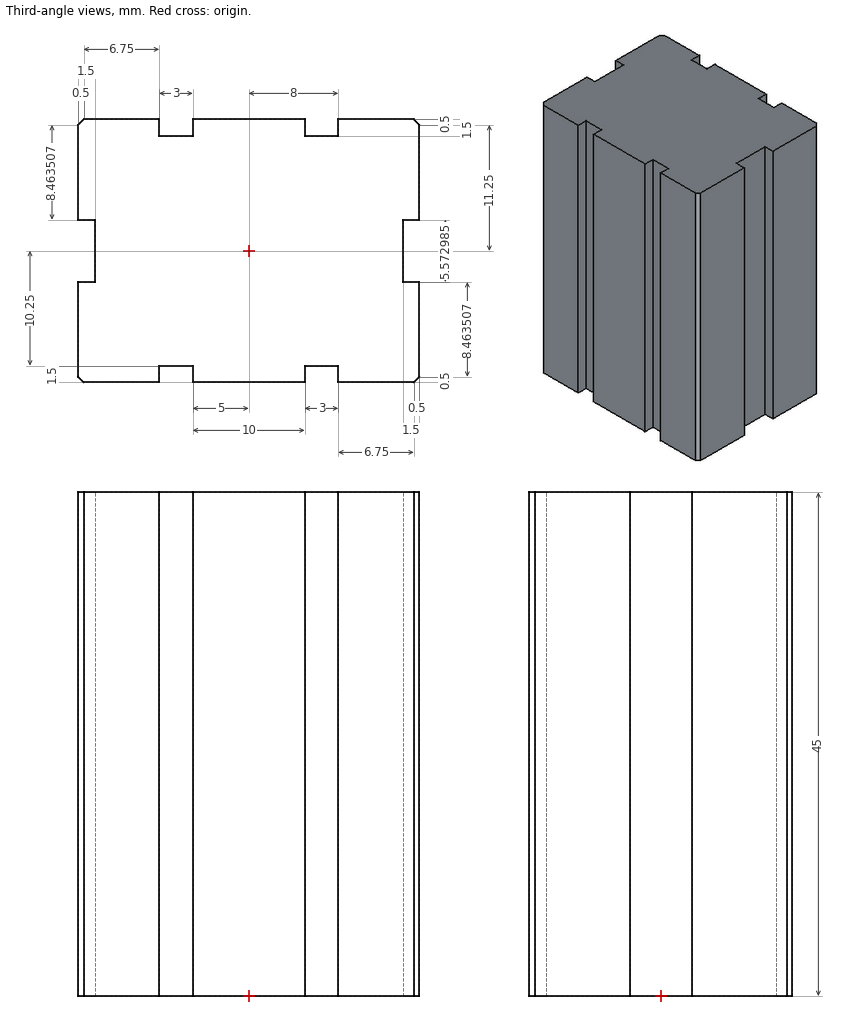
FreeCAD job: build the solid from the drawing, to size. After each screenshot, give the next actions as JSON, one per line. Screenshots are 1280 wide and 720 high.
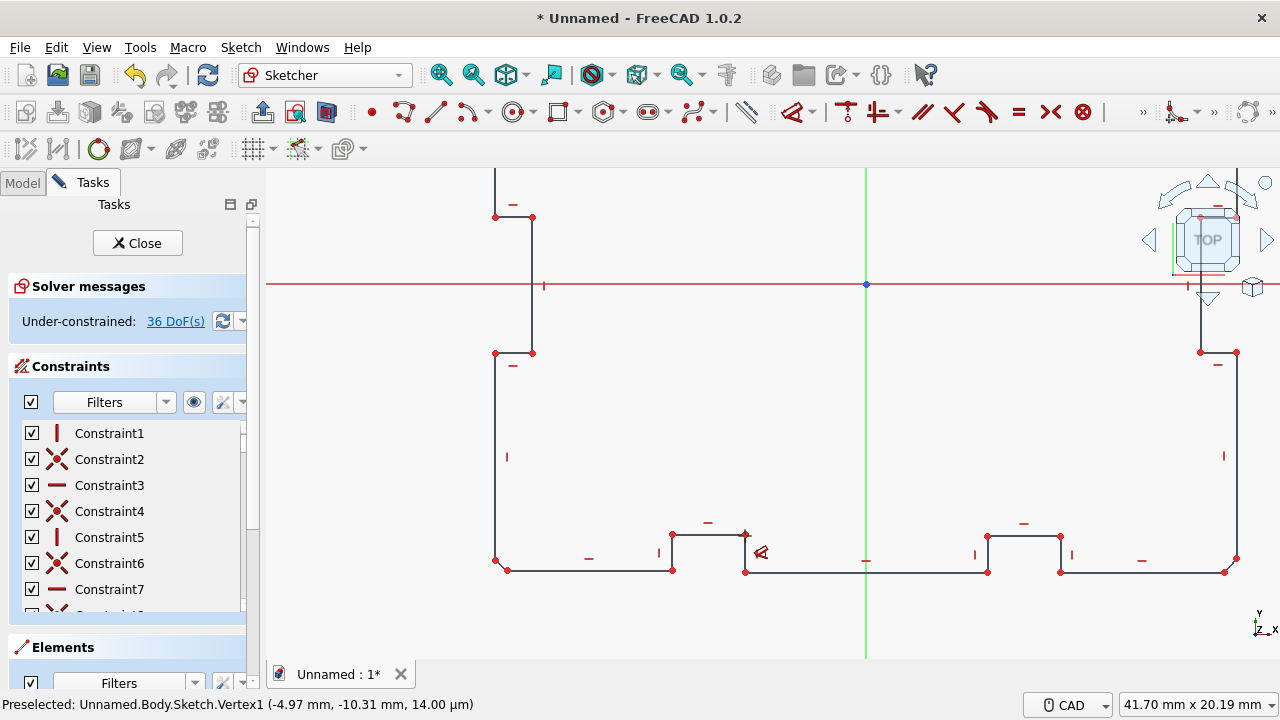
{"action": "left_click", "coordinate": [1010, 536]}
{"action": "left_click", "coordinate": [1024, 570]}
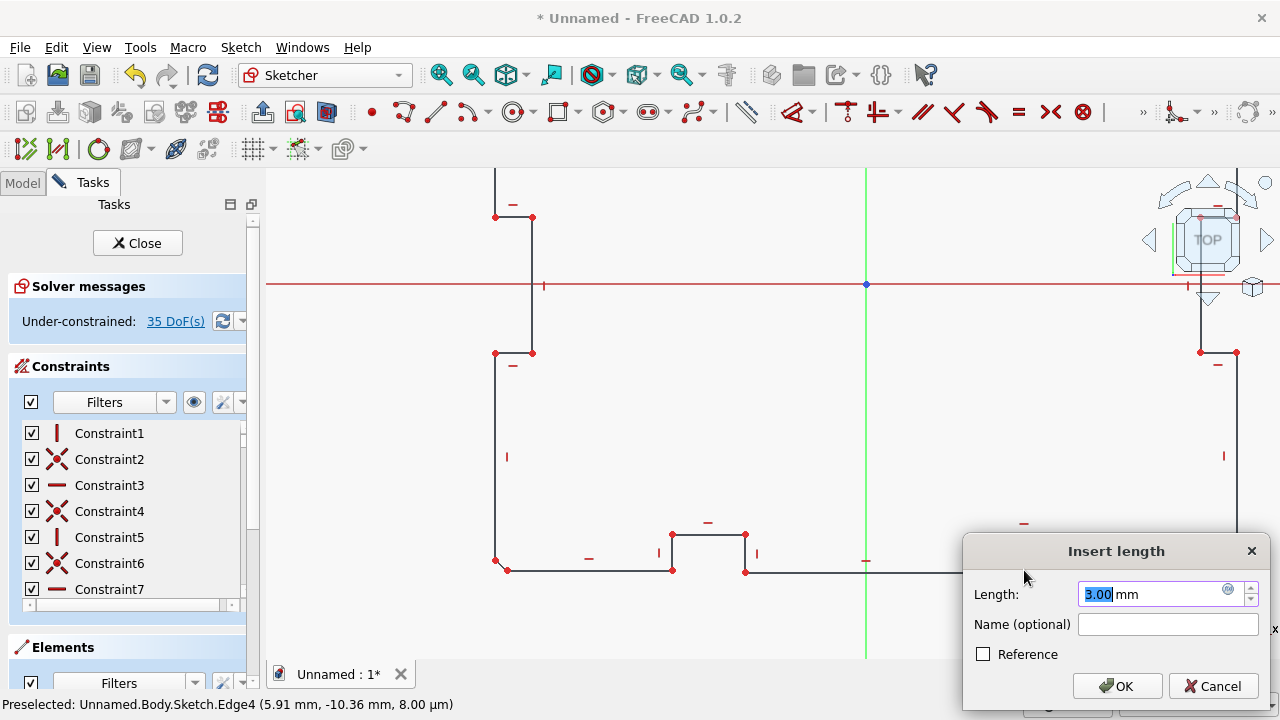
{"action": "type", "text": "3"}
{"action": "key", "text": "Return"}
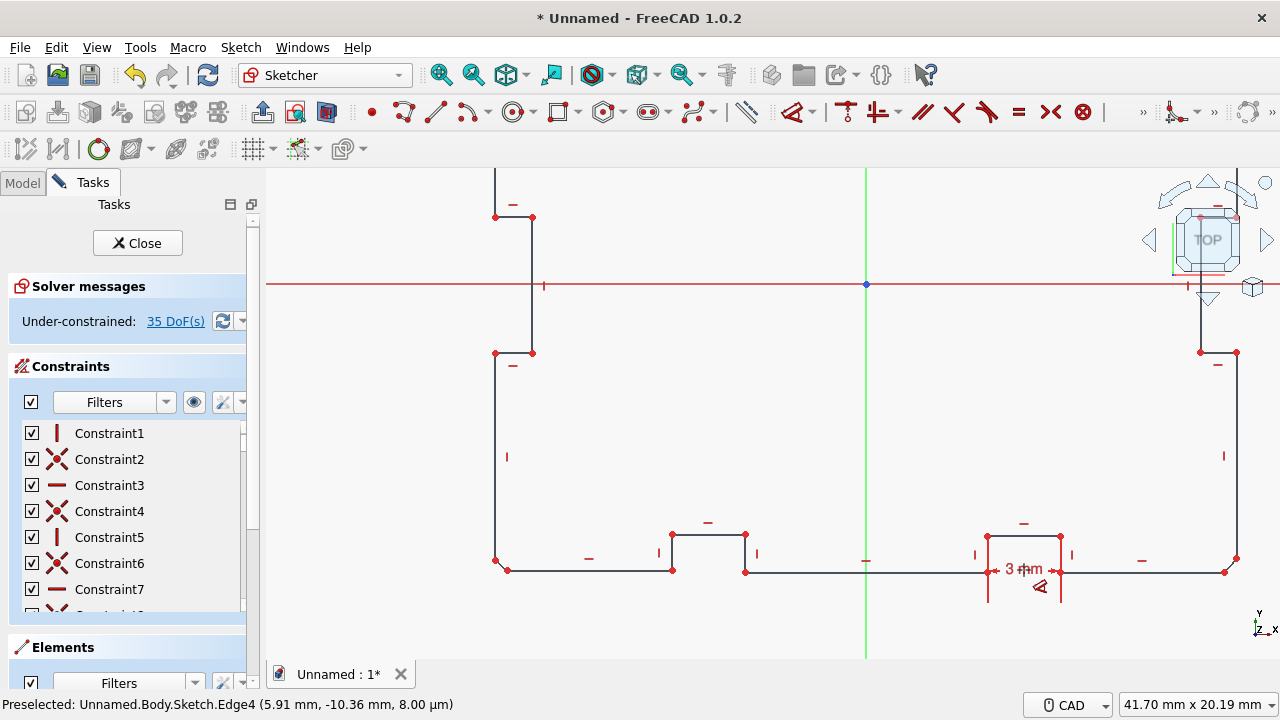
{"action": "scroll", "coordinate": [508, 571], "scroll_direction": "down", "scroll_amount": 3}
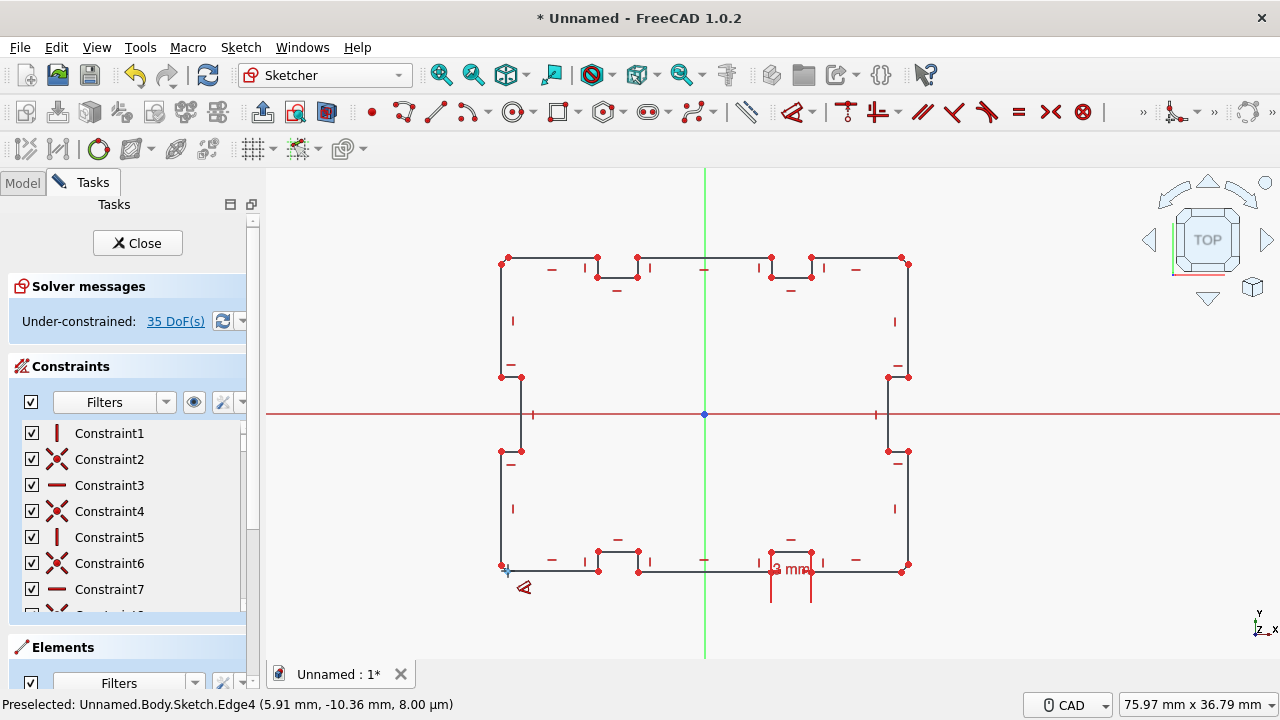
{"action": "left_click", "coordinate": [800, 278]}
{"action": "left_click", "coordinate": [792, 244]}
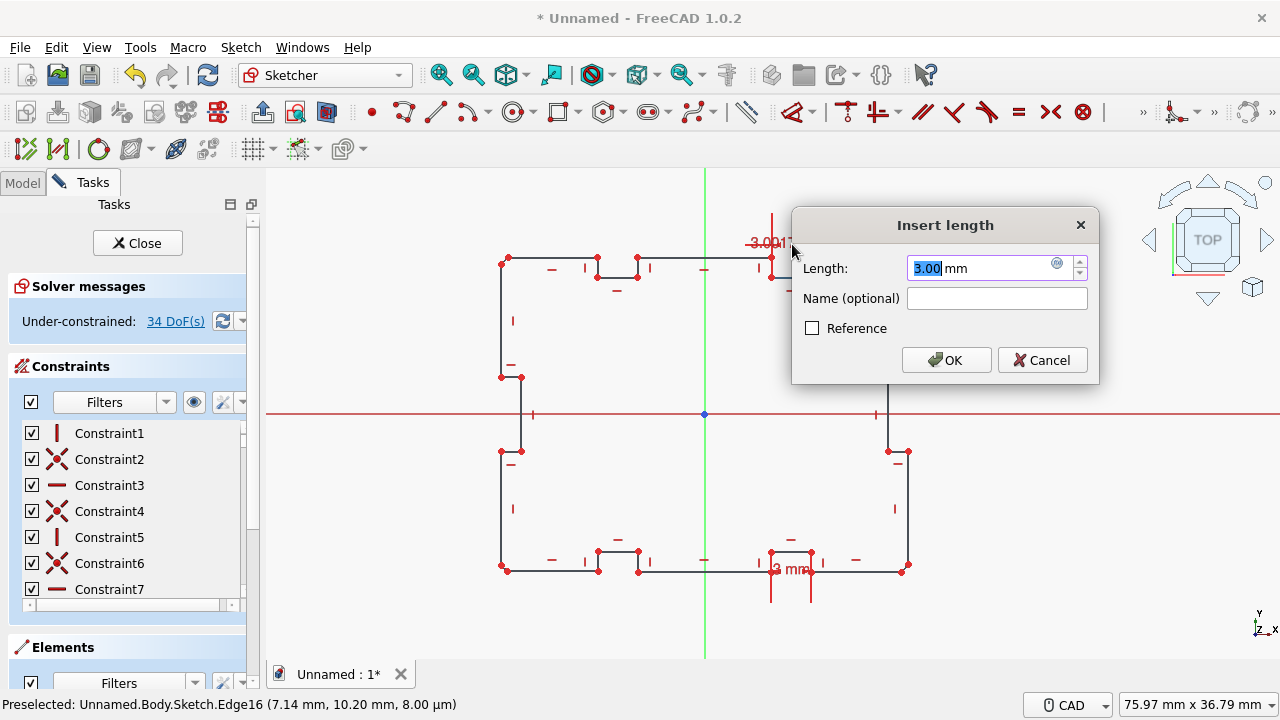
{"action": "type", "text": "3"}
{"action": "key", "text": "Return"}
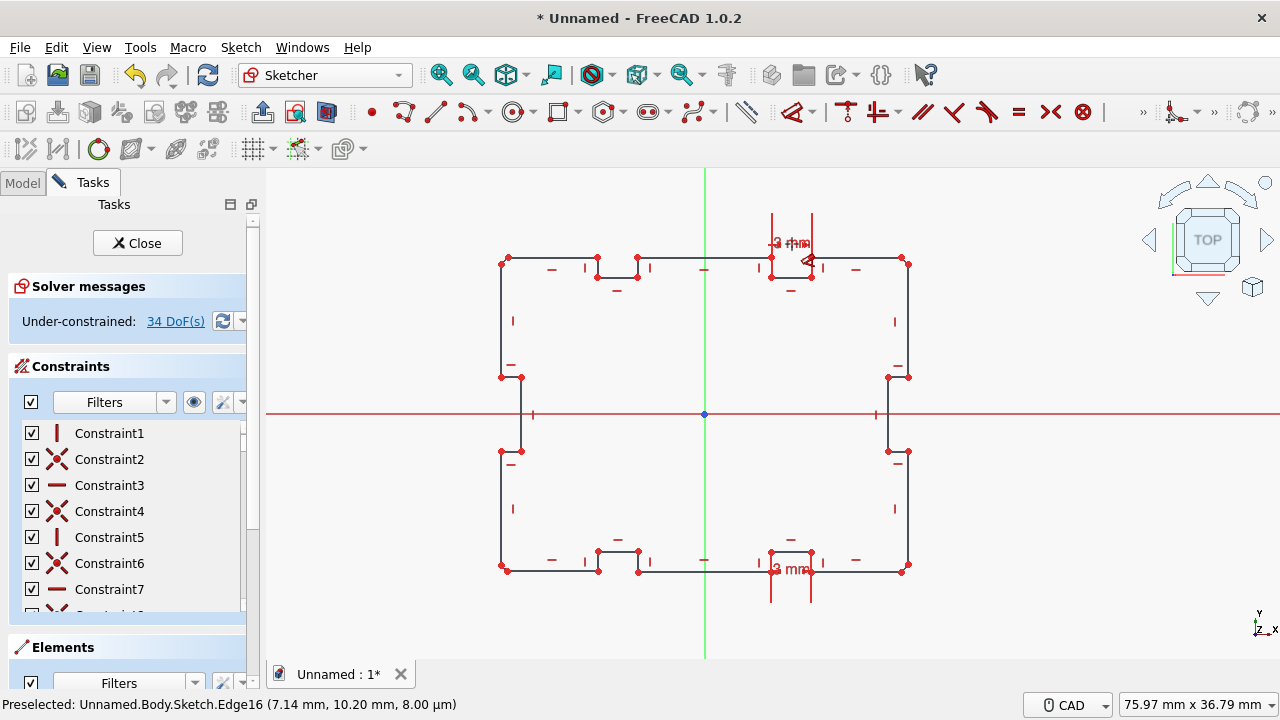
{"action": "left_click", "coordinate": [626, 278]}
{"action": "left_click", "coordinate": [618, 244]}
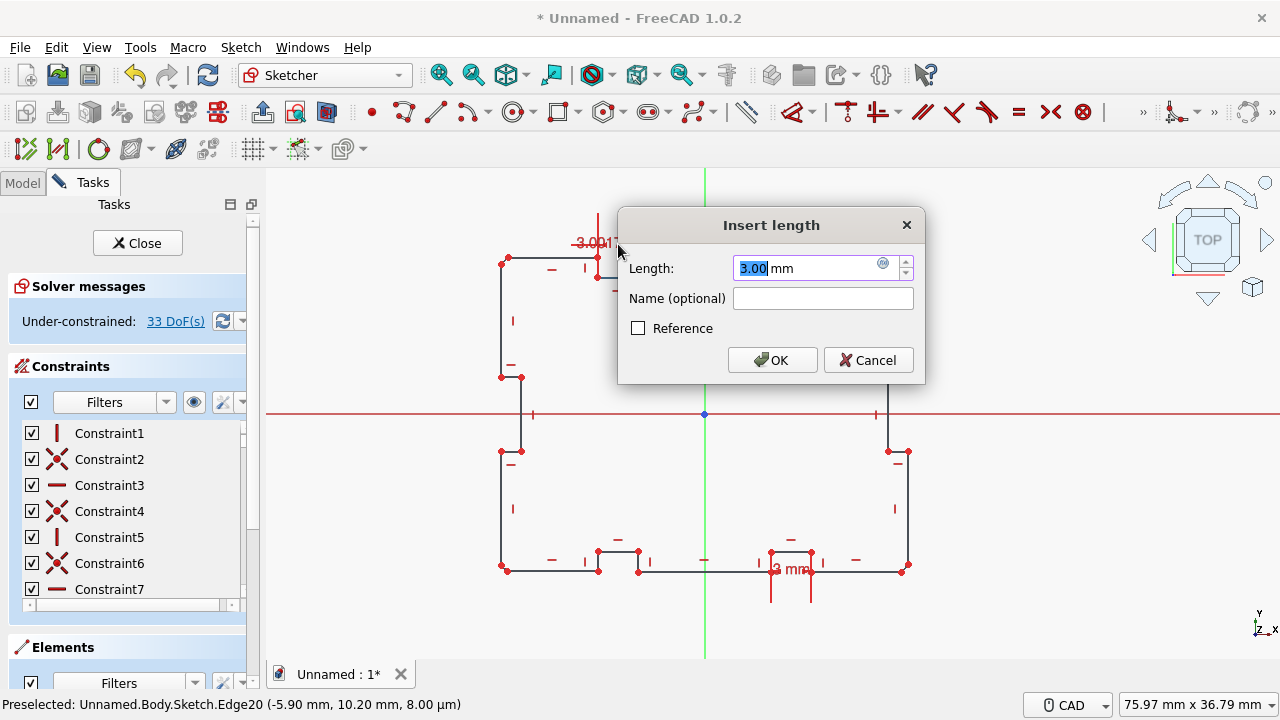
{"action": "type", "text": "3"}
{"action": "key", "text": "Return"}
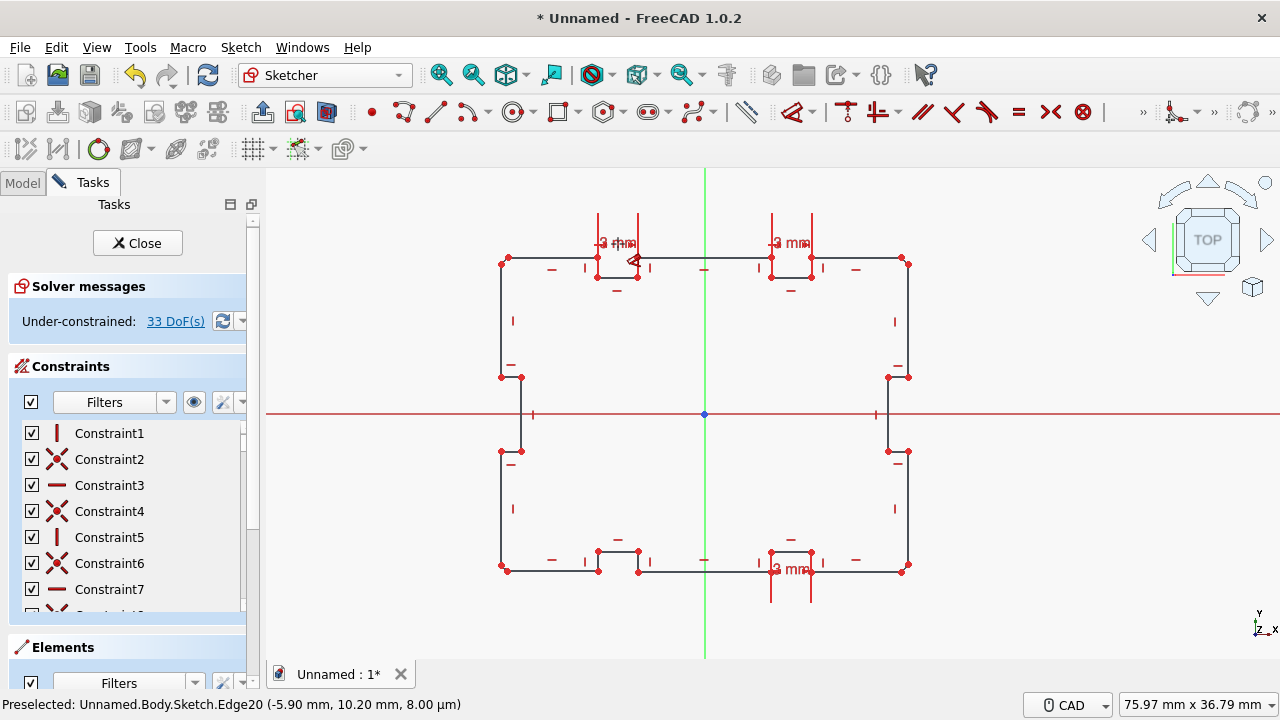
{"action": "left_click", "coordinate": [610, 552]}
{"action": "left_click", "coordinate": [618, 586]}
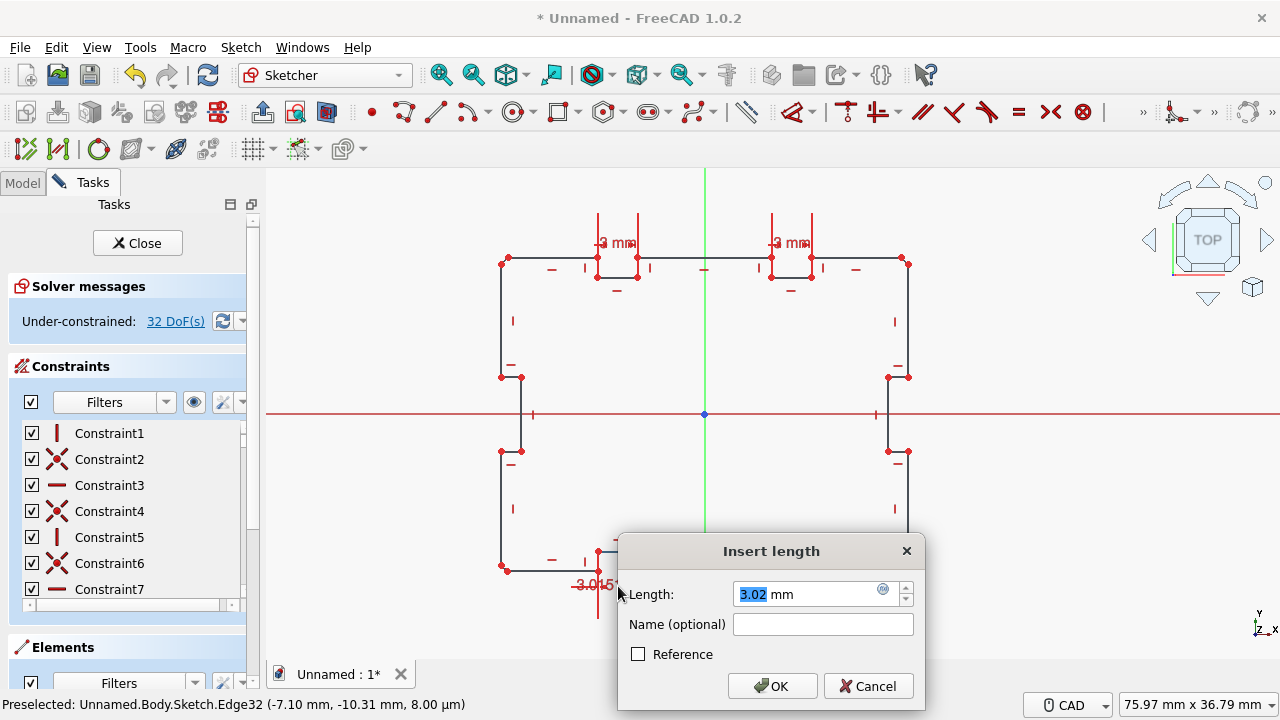
{"action": "type", "text": "3"}
{"action": "key", "text": "Return"}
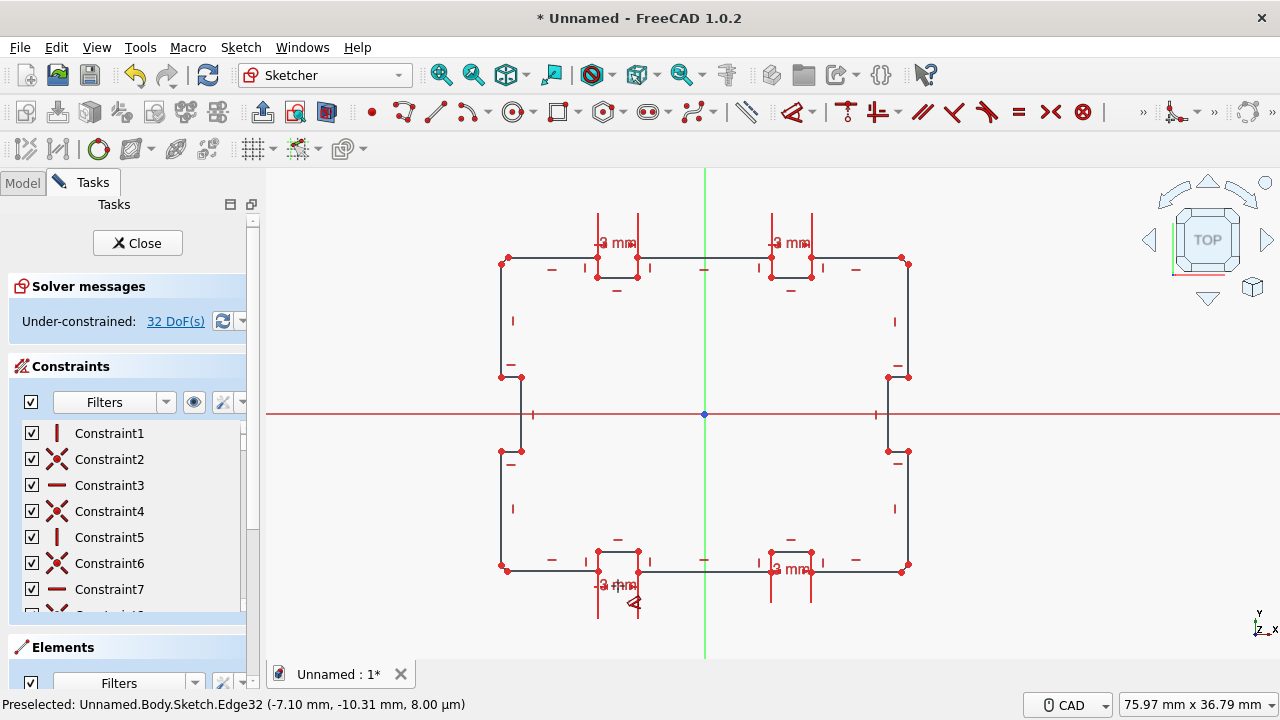
{"action": "left_click", "coordinate": [678, 572]}
{"action": "left_click", "coordinate": [674, 606]}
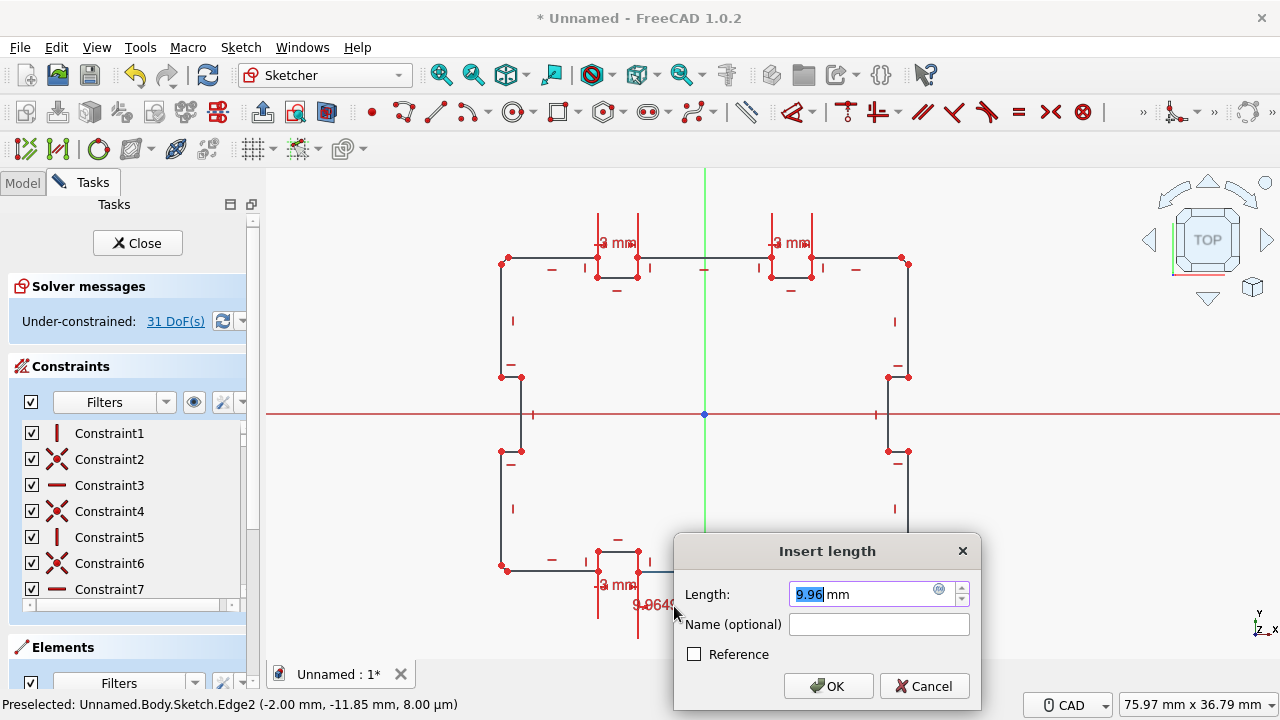
{"action": "type", "text": "10"}
{"action": "key", "text": "Return"}